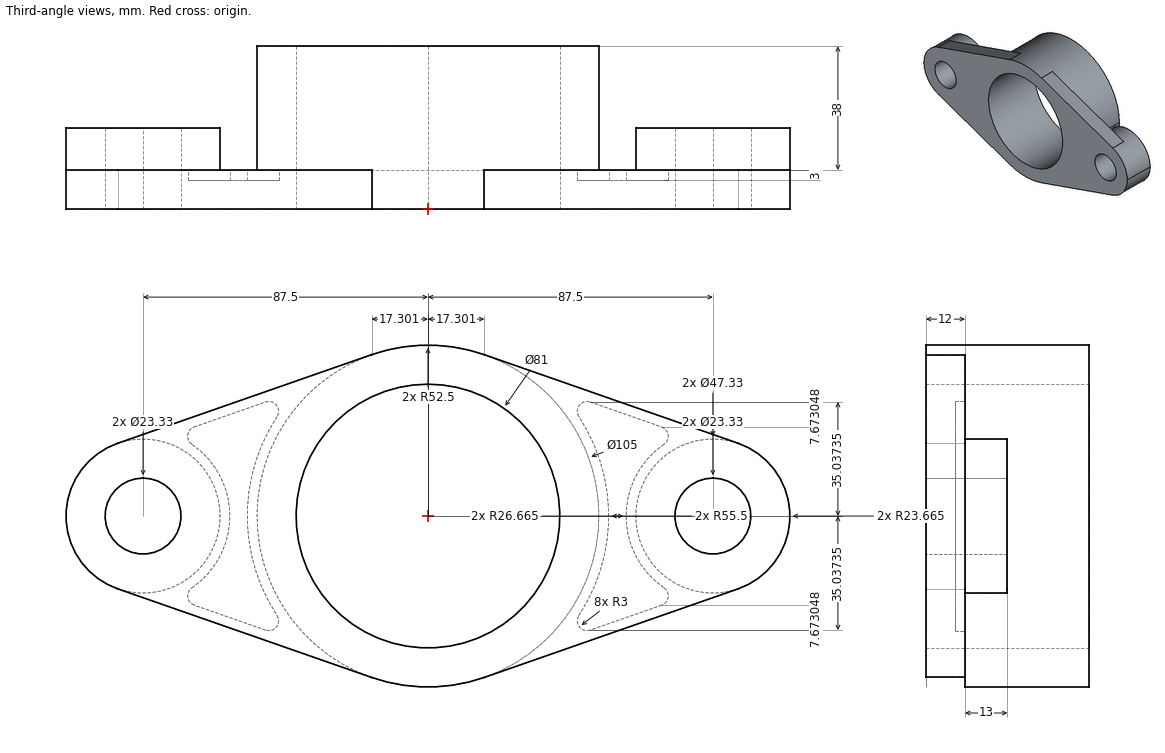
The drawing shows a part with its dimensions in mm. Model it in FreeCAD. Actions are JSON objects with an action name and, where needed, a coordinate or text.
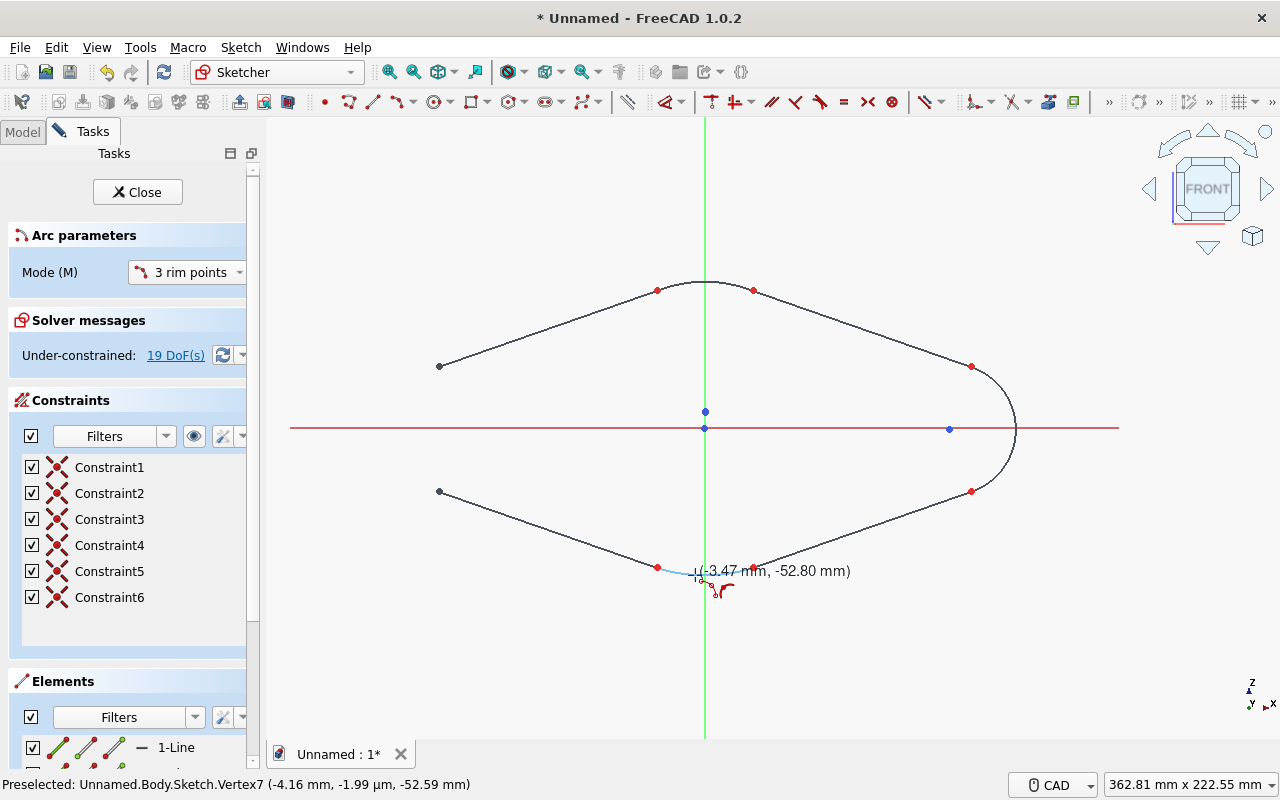
{"action": "left_click", "coordinate": [439, 492]}
{"action": "left_click", "coordinate": [439, 367]}
{"action": "left_click", "coordinate": [396, 412]}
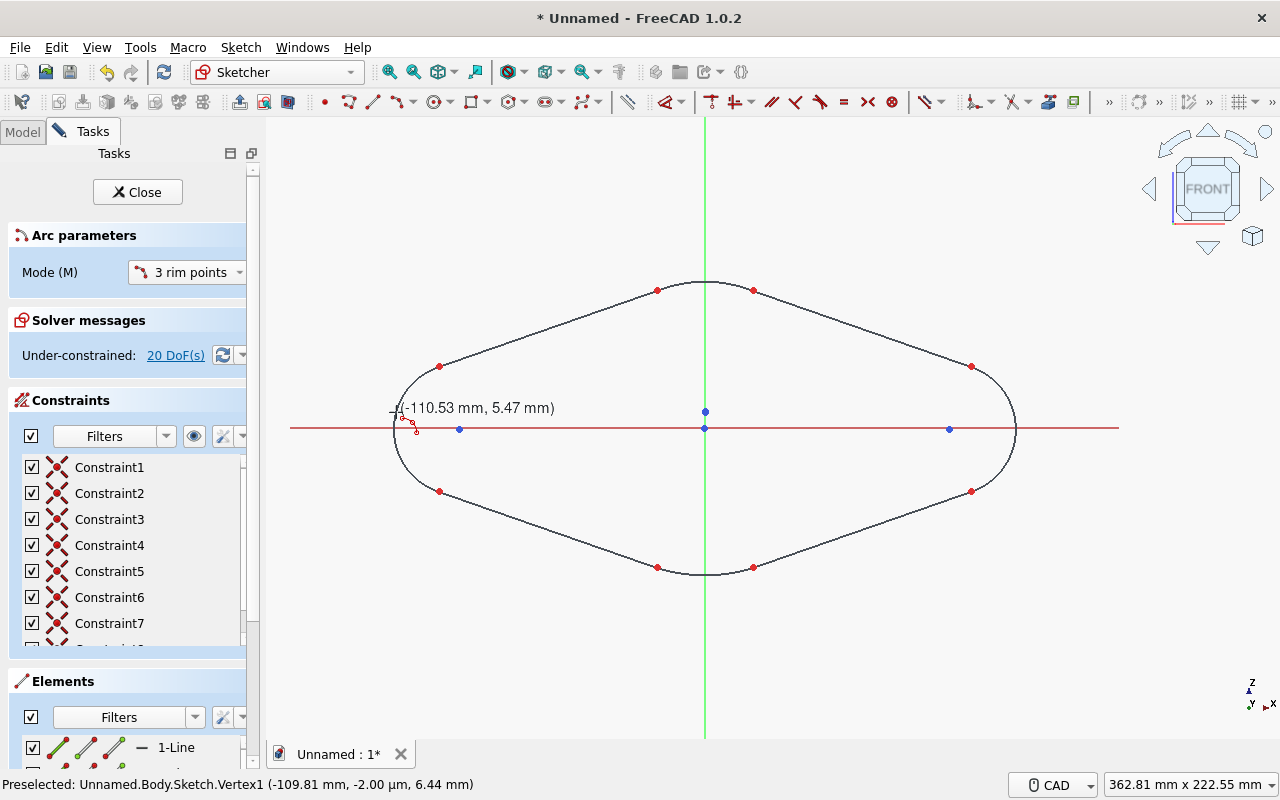
{"action": "left_click", "coordinate": [434, 102]}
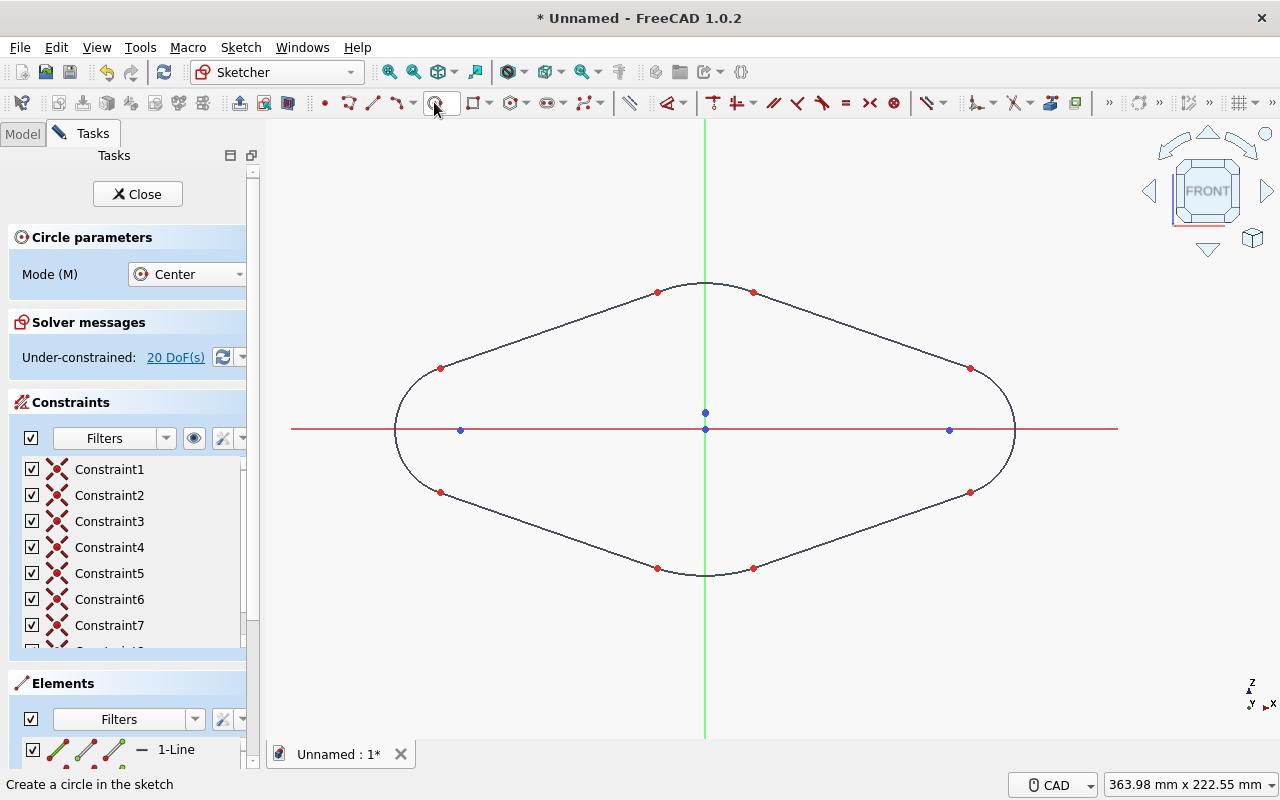
{"action": "left_click", "coordinate": [461, 429]}
{"action": "mouse_move", "coordinate": [484, 406]}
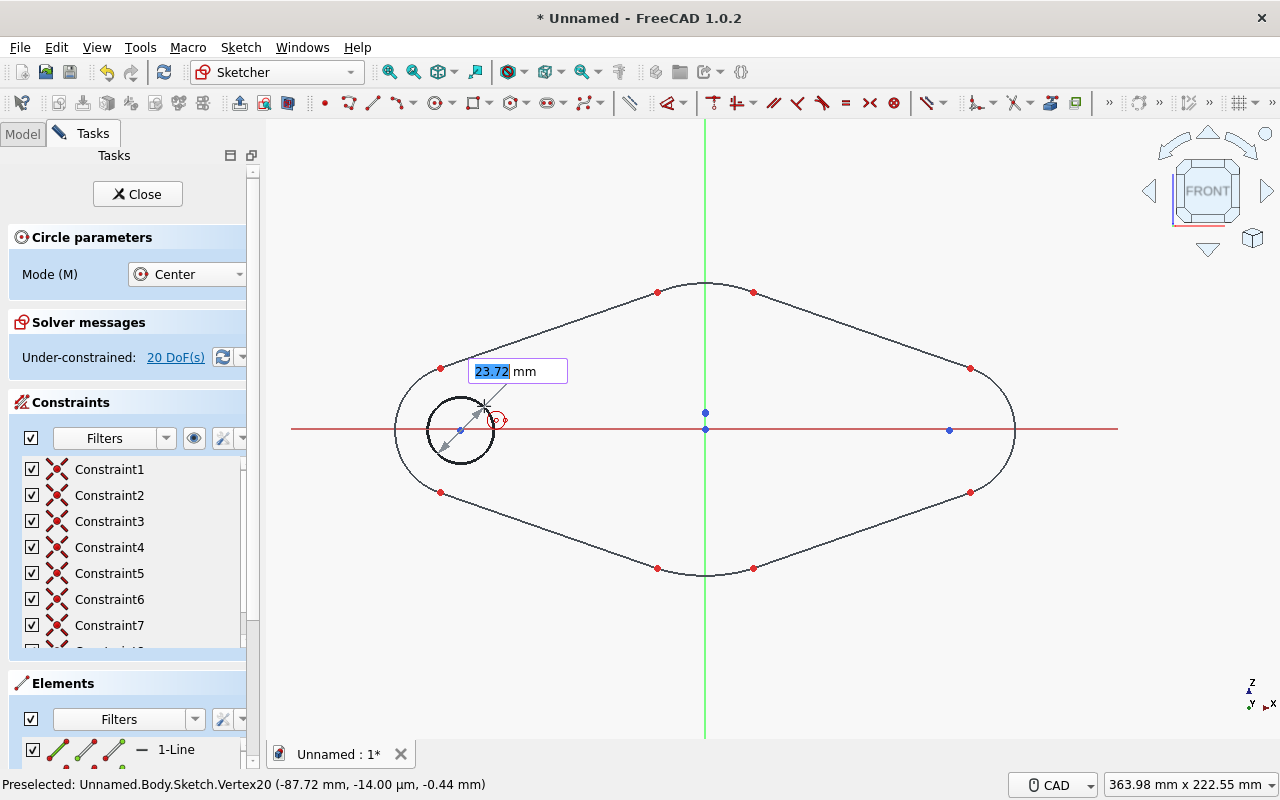
{"action": "type", "text": "23.33"}
{"action": "key", "text": "Return"}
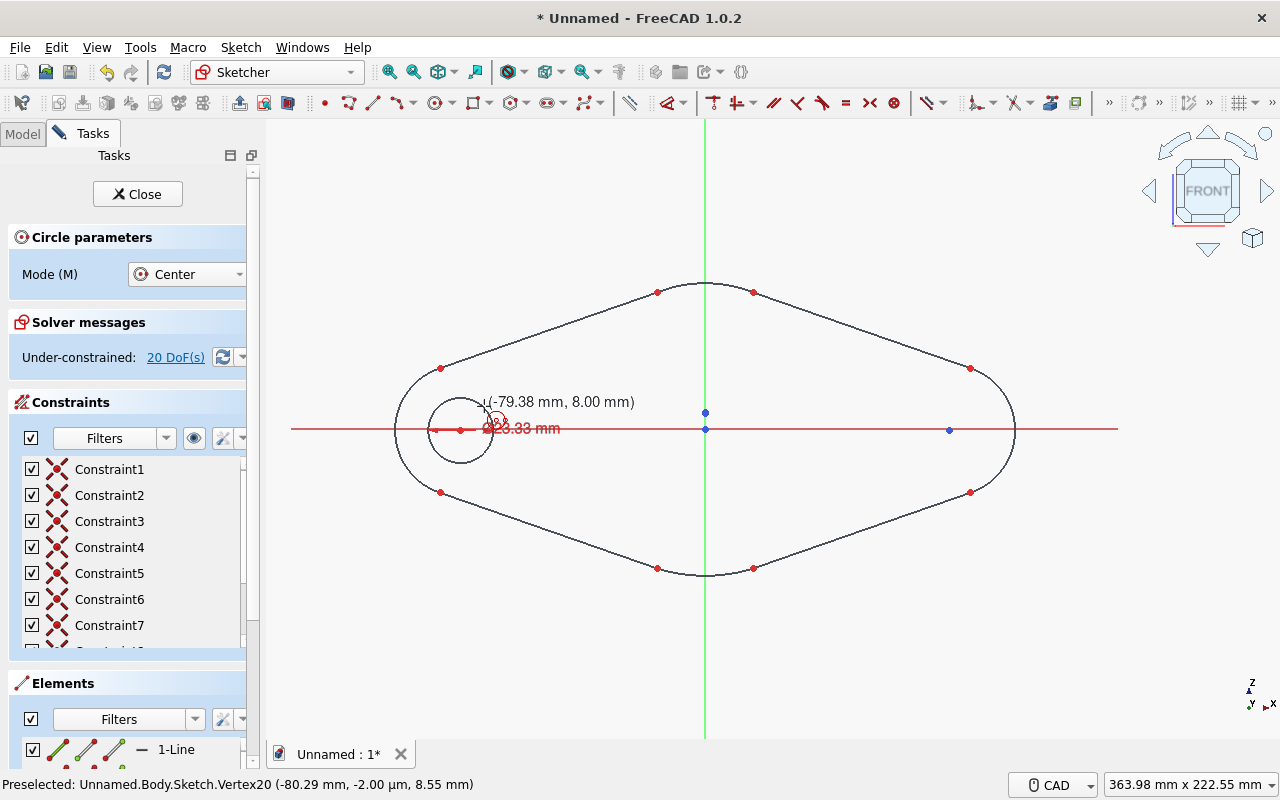
{"action": "left_click", "coordinate": [705, 429]}
{"action": "mouse_move", "coordinate": [785, 349]}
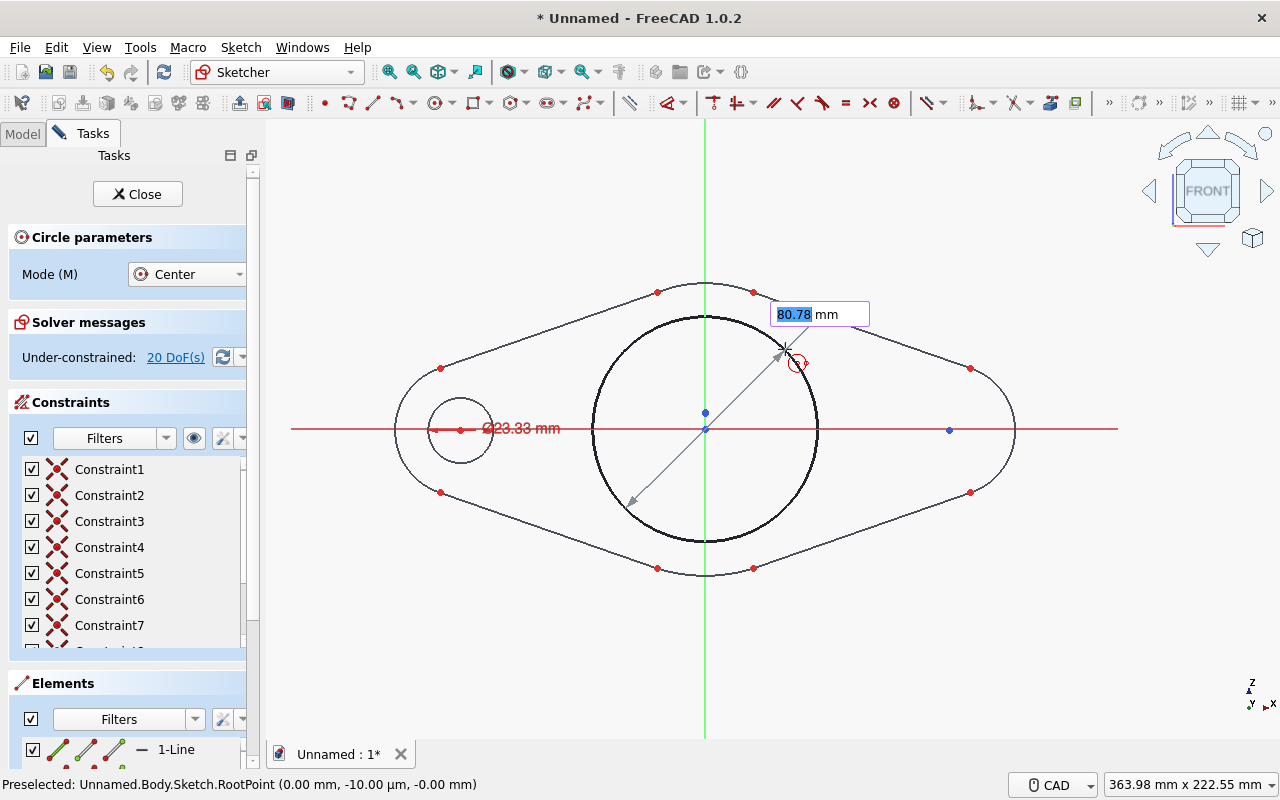
{"action": "type", "text": "81"}
{"action": "key", "text": "Return"}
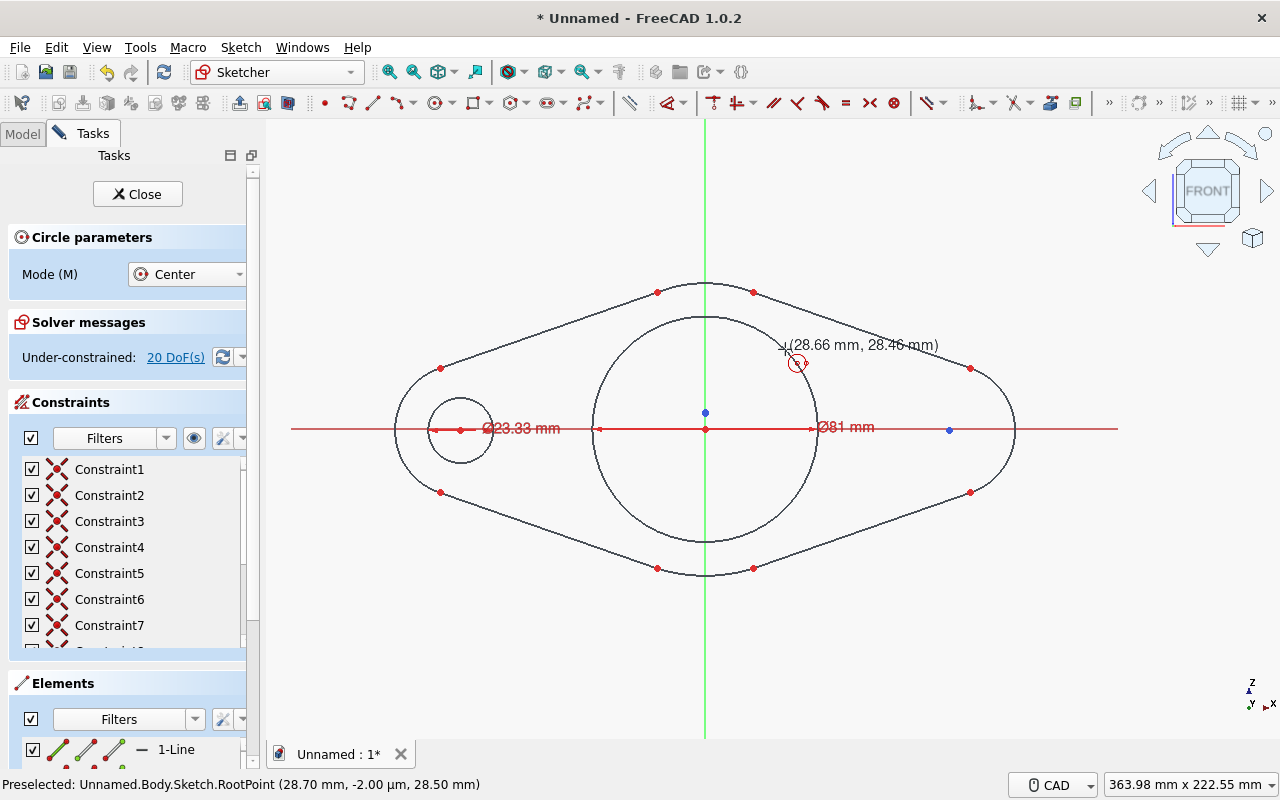
{"action": "left_click", "coordinate": [949, 429]}
{"action": "mouse_move", "coordinate": [972, 406]}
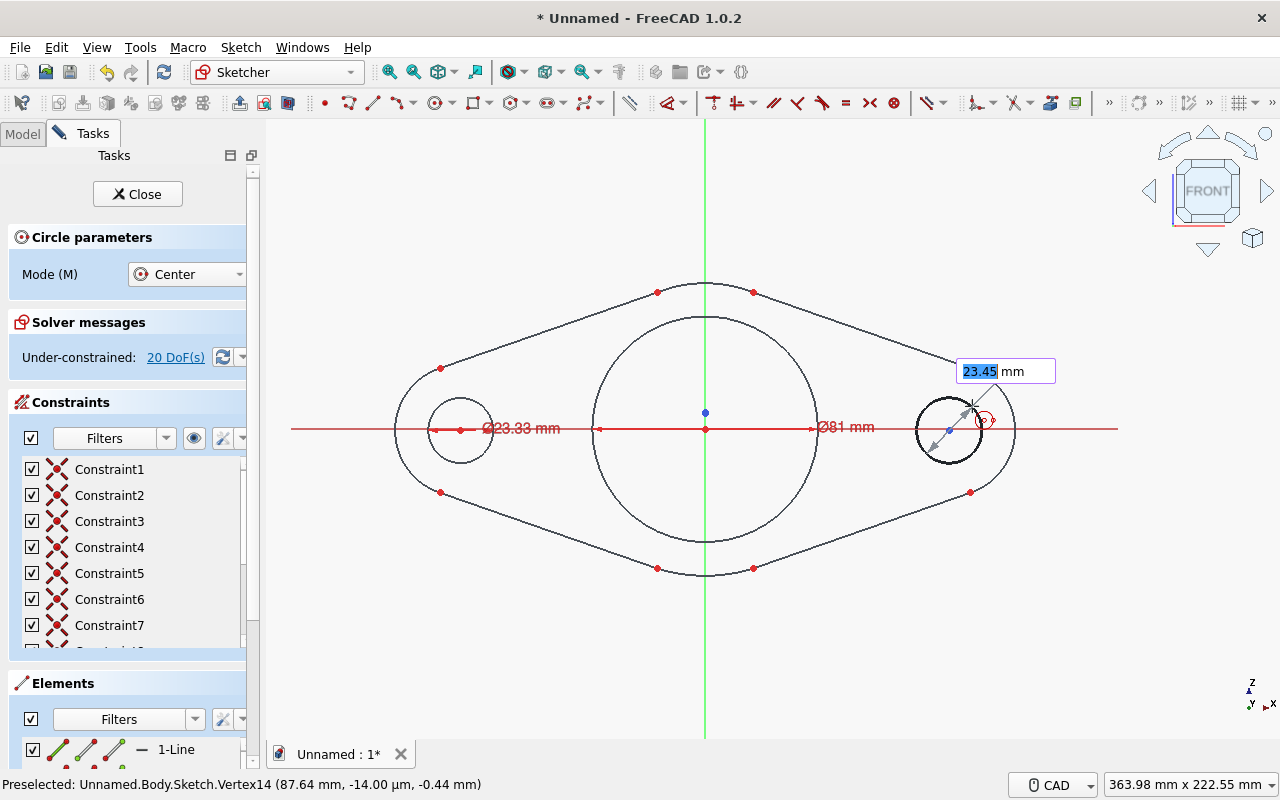
{"action": "type", "text": "23.33"}
{"action": "key", "text": "Return"}
{"action": "key", "text": "Escape"}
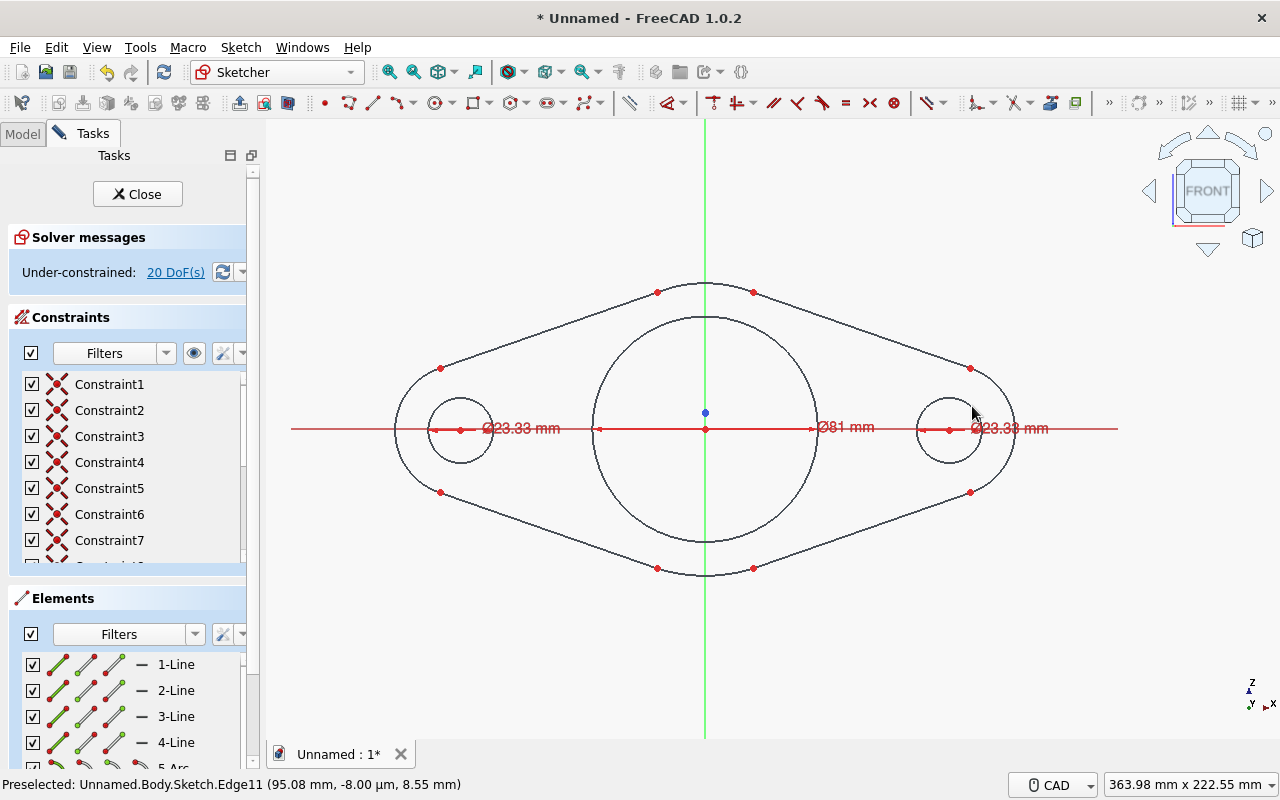
{"action": "left_click", "coordinate": [505, 345]}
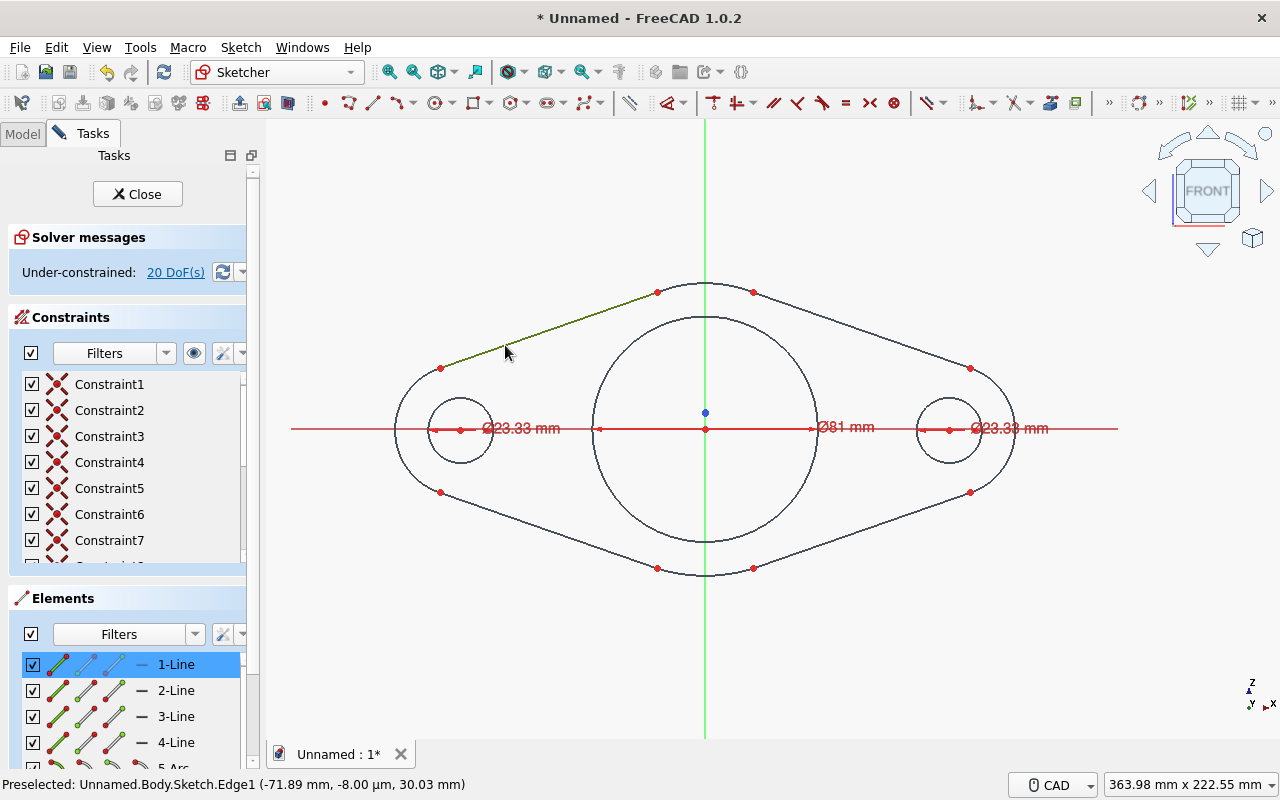
{"action": "left_click", "coordinate": [403, 399]}